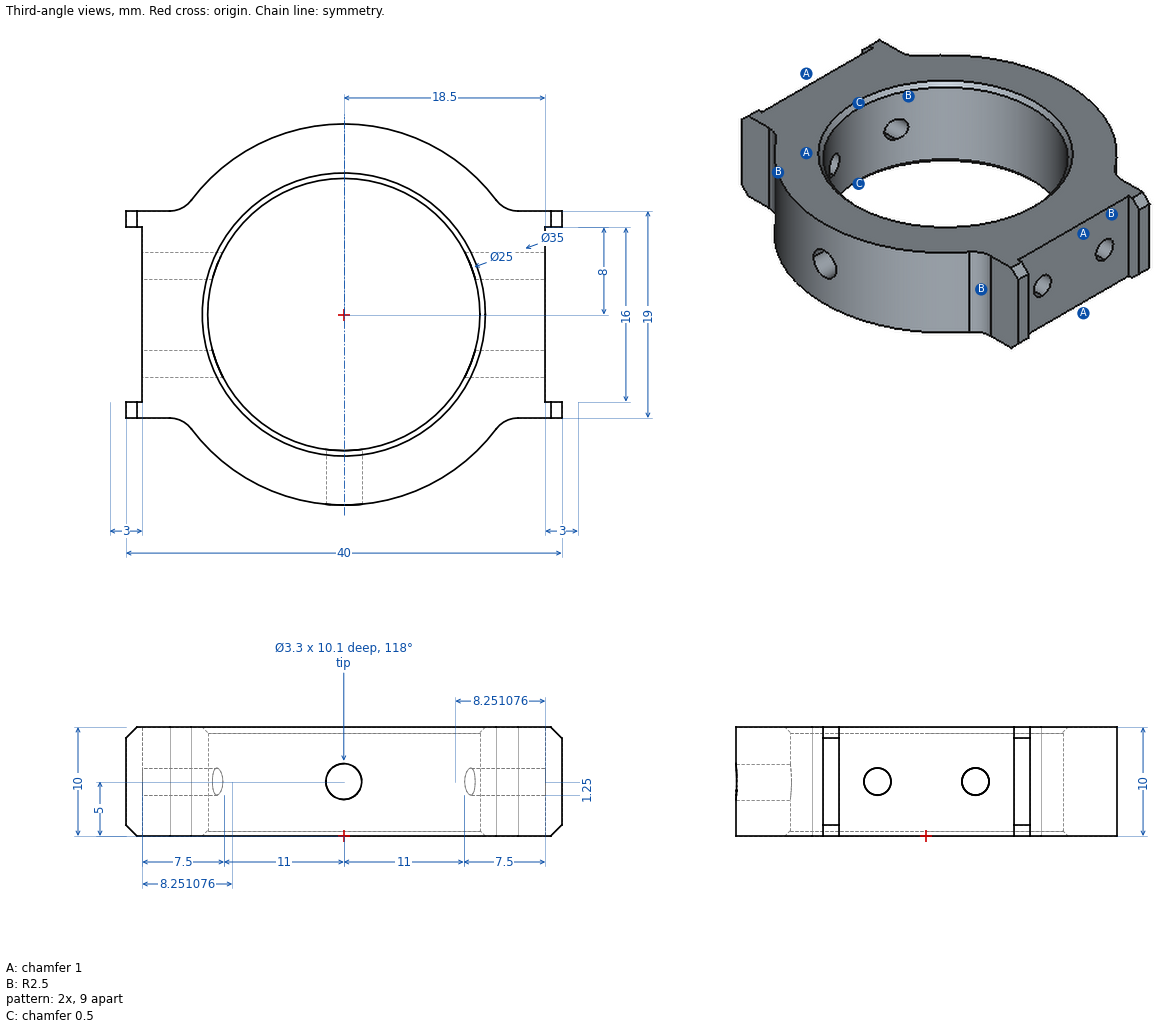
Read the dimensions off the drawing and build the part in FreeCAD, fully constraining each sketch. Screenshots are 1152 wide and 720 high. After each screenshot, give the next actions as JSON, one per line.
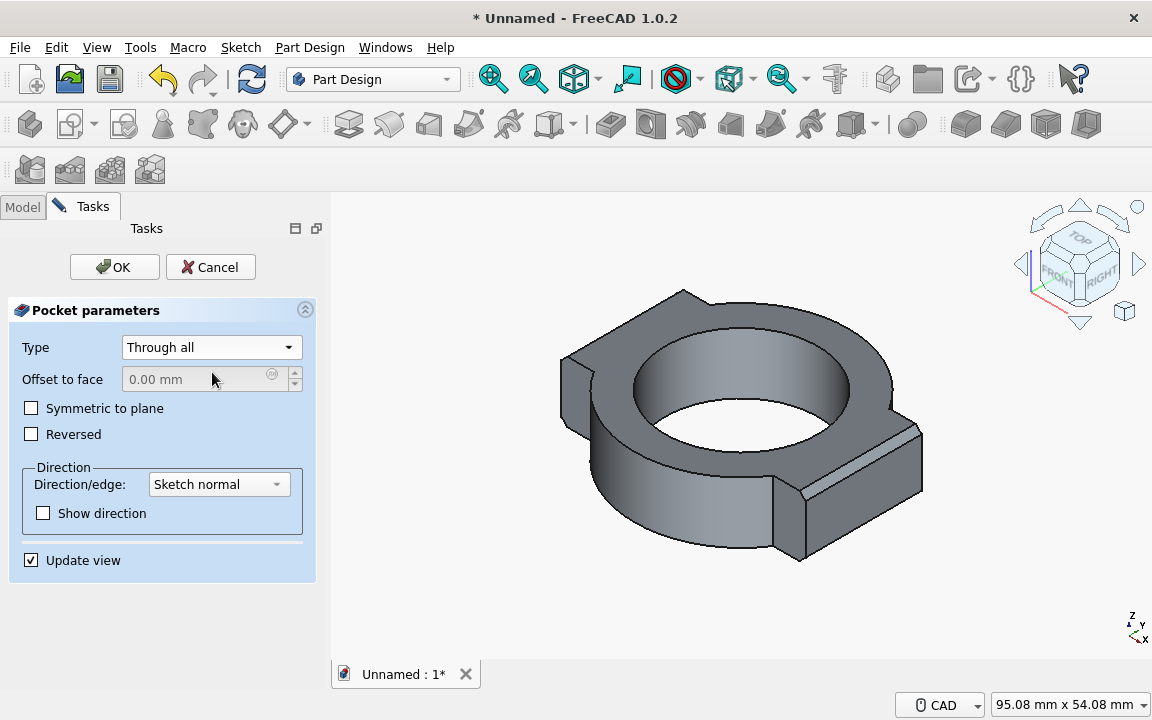
{"action": "left_click", "coordinate": [115, 267]}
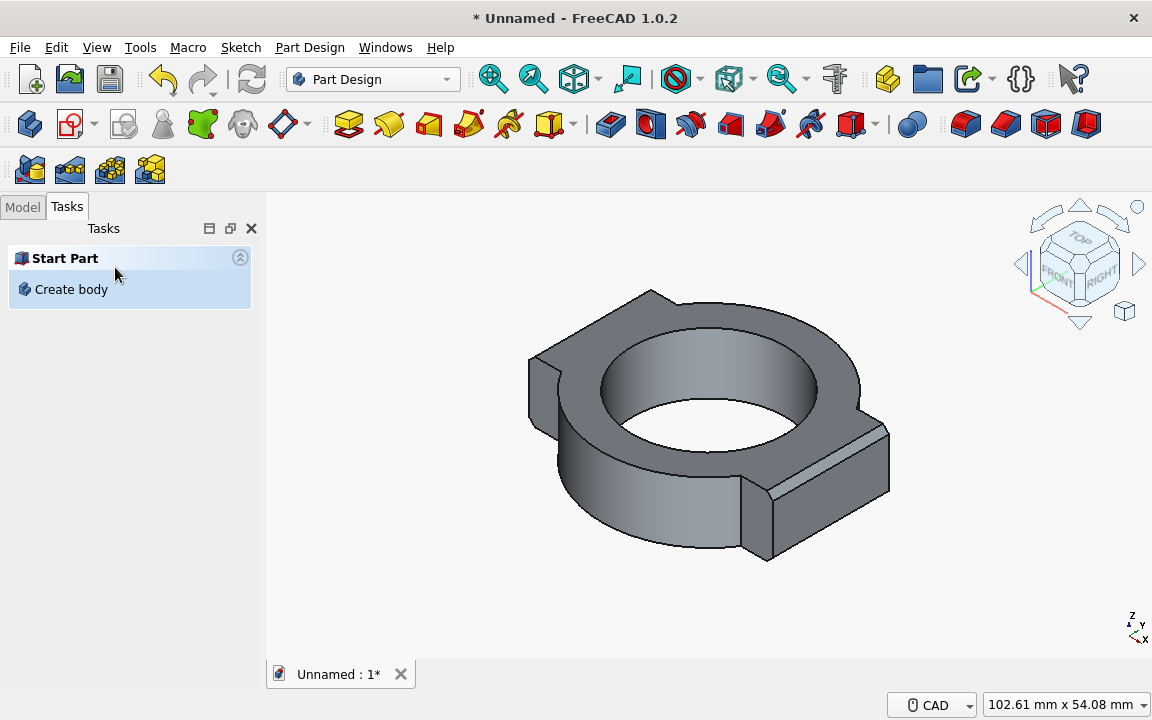
{"action": "left_click", "coordinate": [839, 429]}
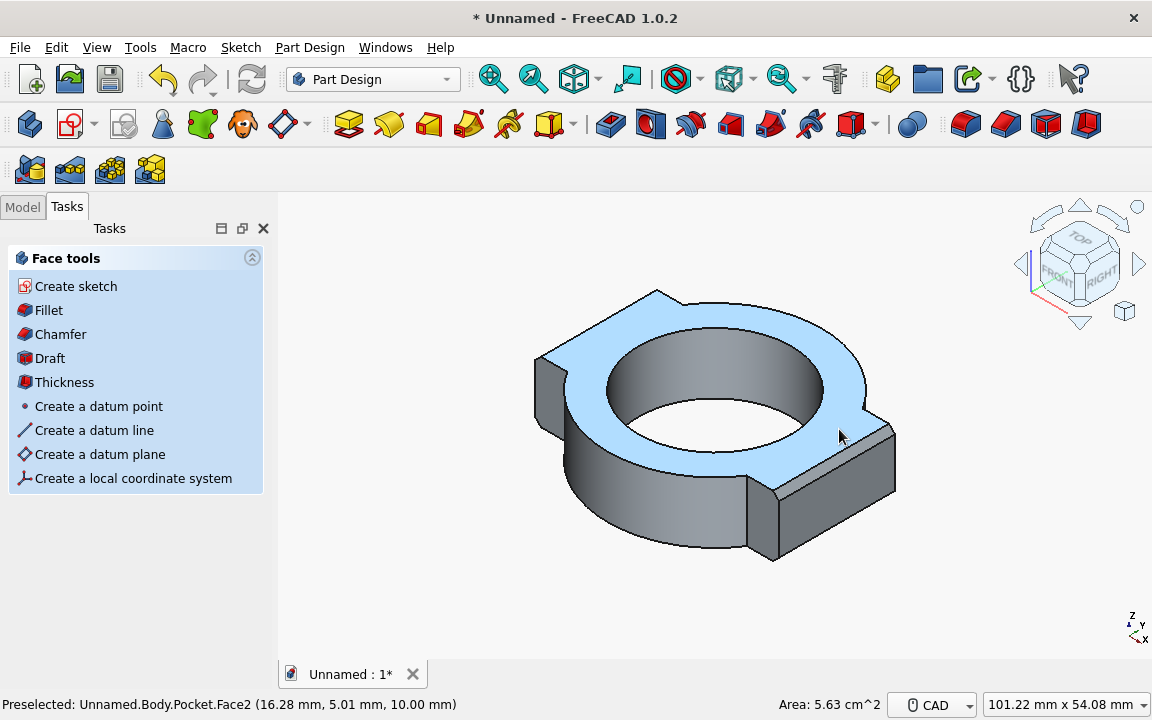
{"action": "left_click", "coordinate": [70, 124]}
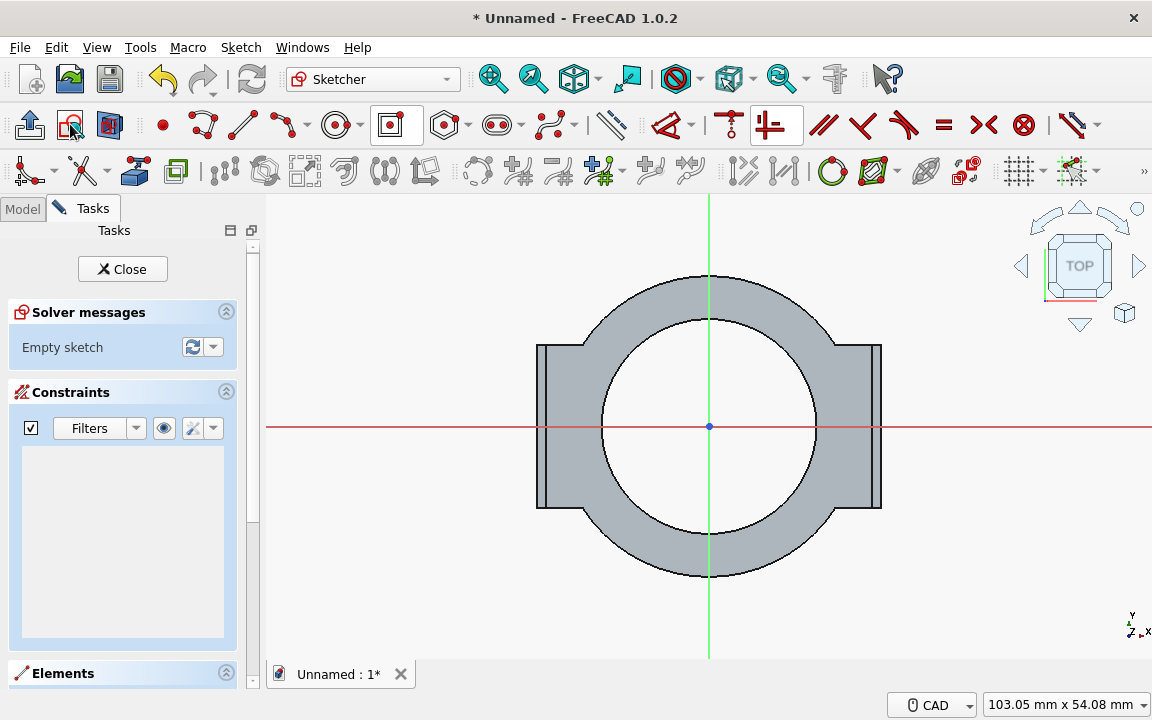
{"action": "left_click", "coordinate": [418, 126]}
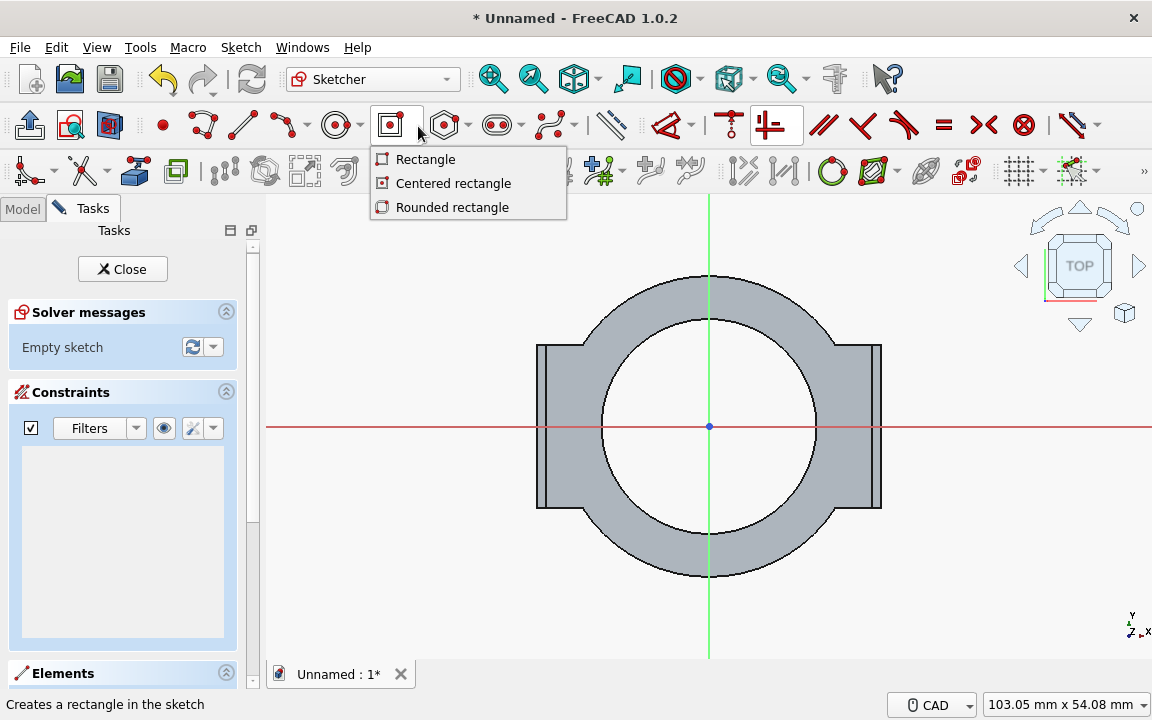
{"action": "left_click", "coordinate": [468, 159]}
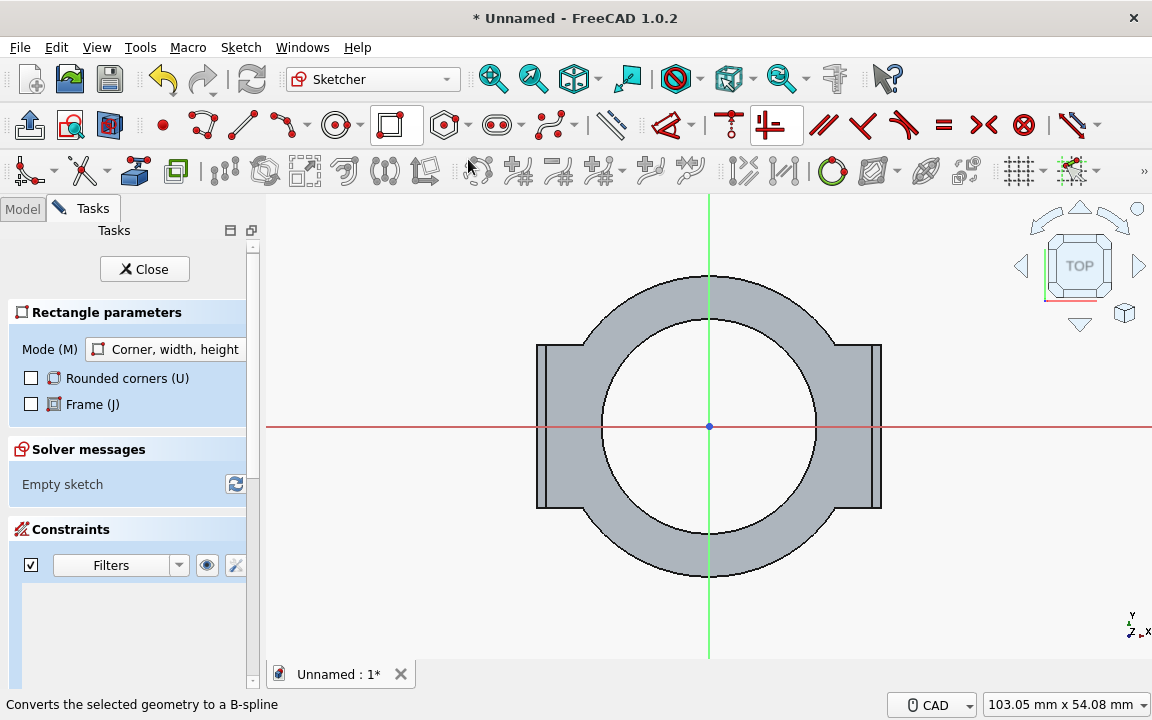
{"action": "left_click", "coordinate": [868, 358]}
{"action": "mouse_move", "coordinate": [894, 495]}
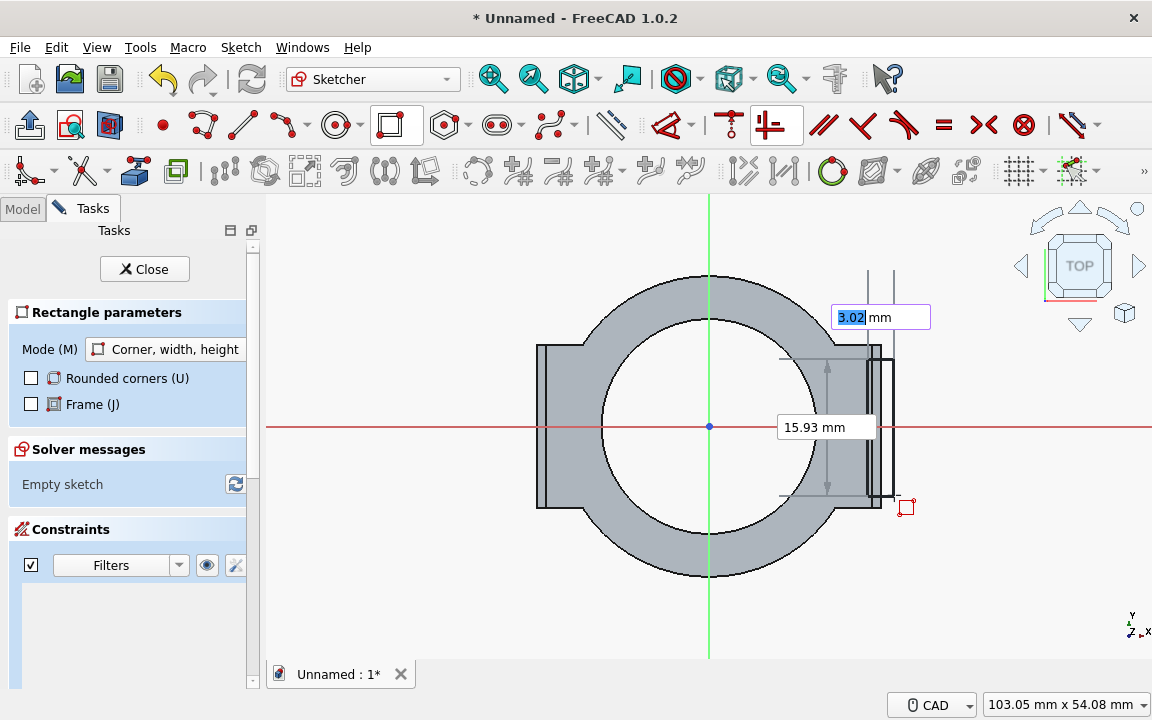
{"action": "type", "text": "3"}
{"action": "key", "text": "Tab"}
{"action": "type", "text": "16"}
{"action": "key", "text": "Return"}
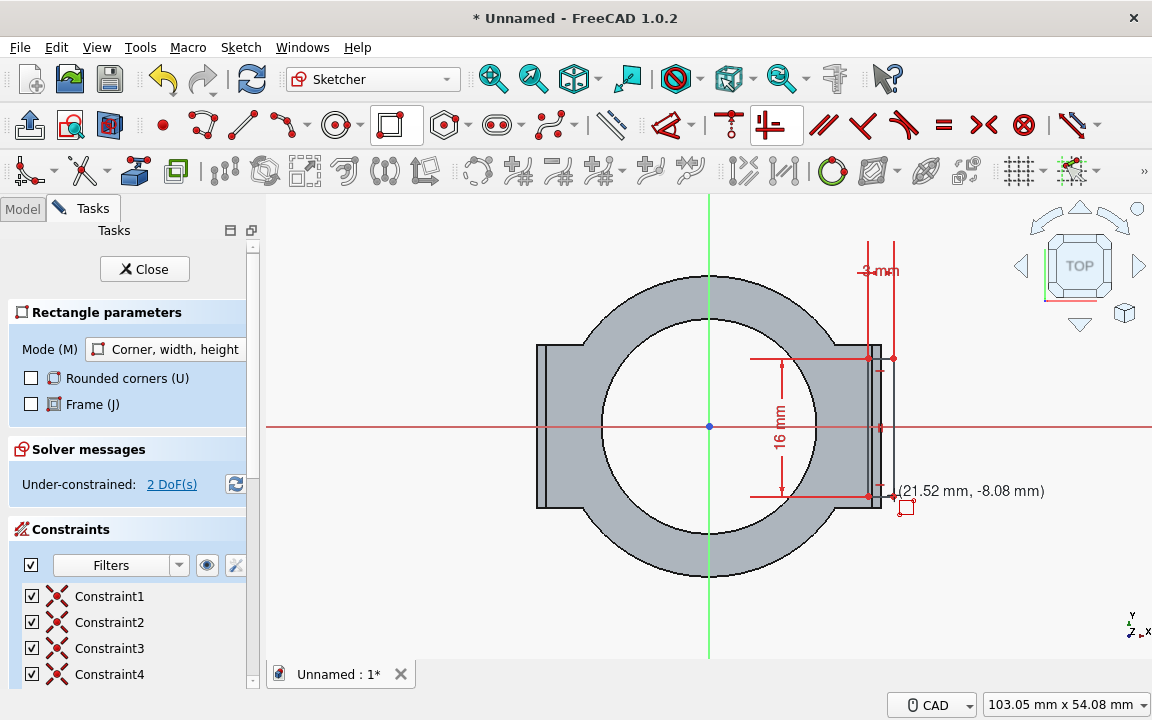
{"action": "left_click", "coordinate": [524, 358]}
{"action": "mouse_move", "coordinate": [550, 495]}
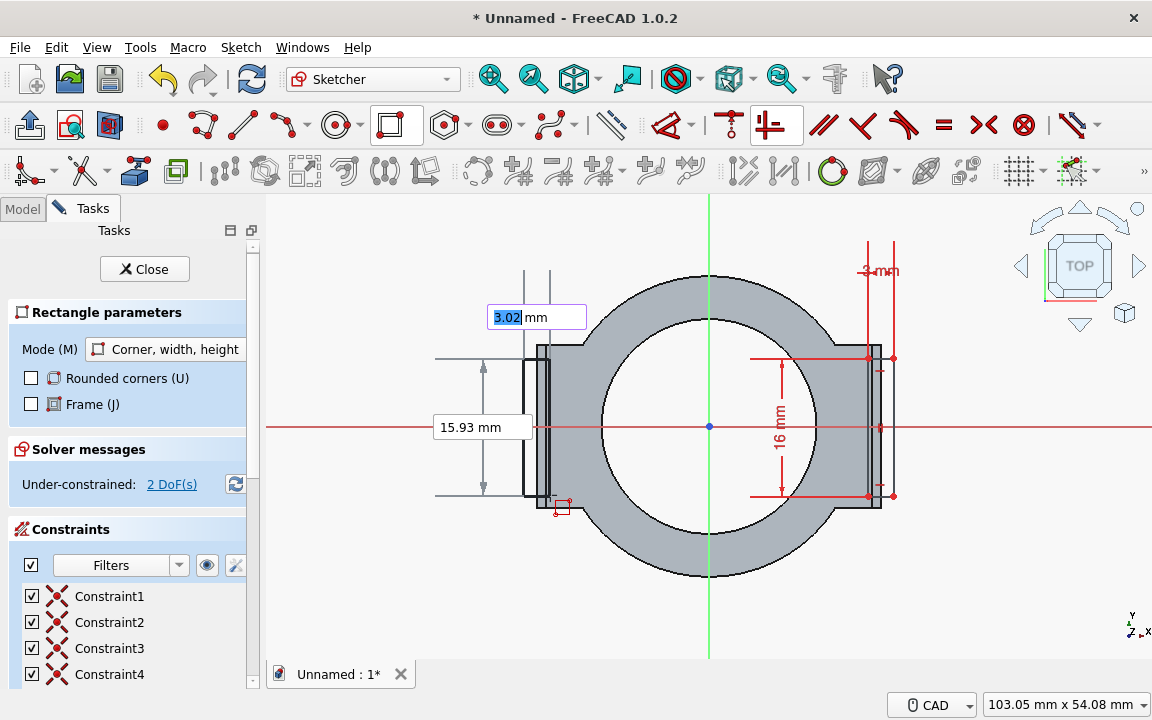
{"action": "type", "text": "3"}
{"action": "key", "text": "Tab"}
{"action": "type", "text": "16"}
{"action": "key", "text": "Return"}
{"action": "key", "text": "Escape"}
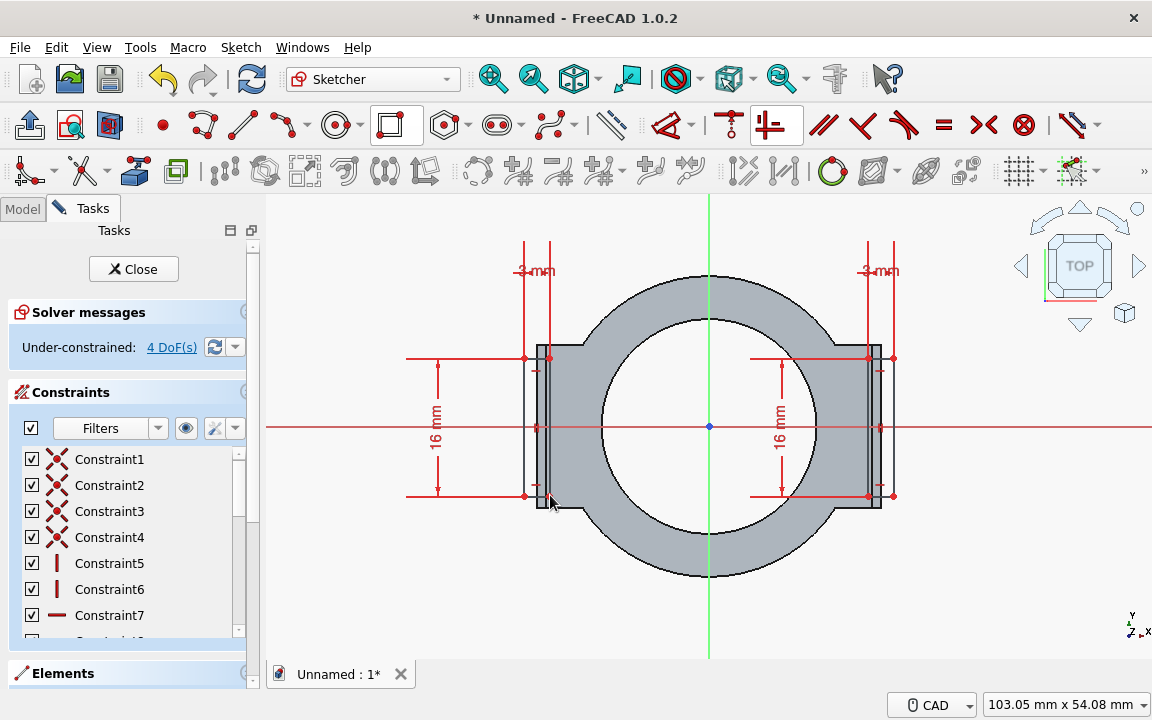
{"action": "left_click", "coordinate": [894, 359]}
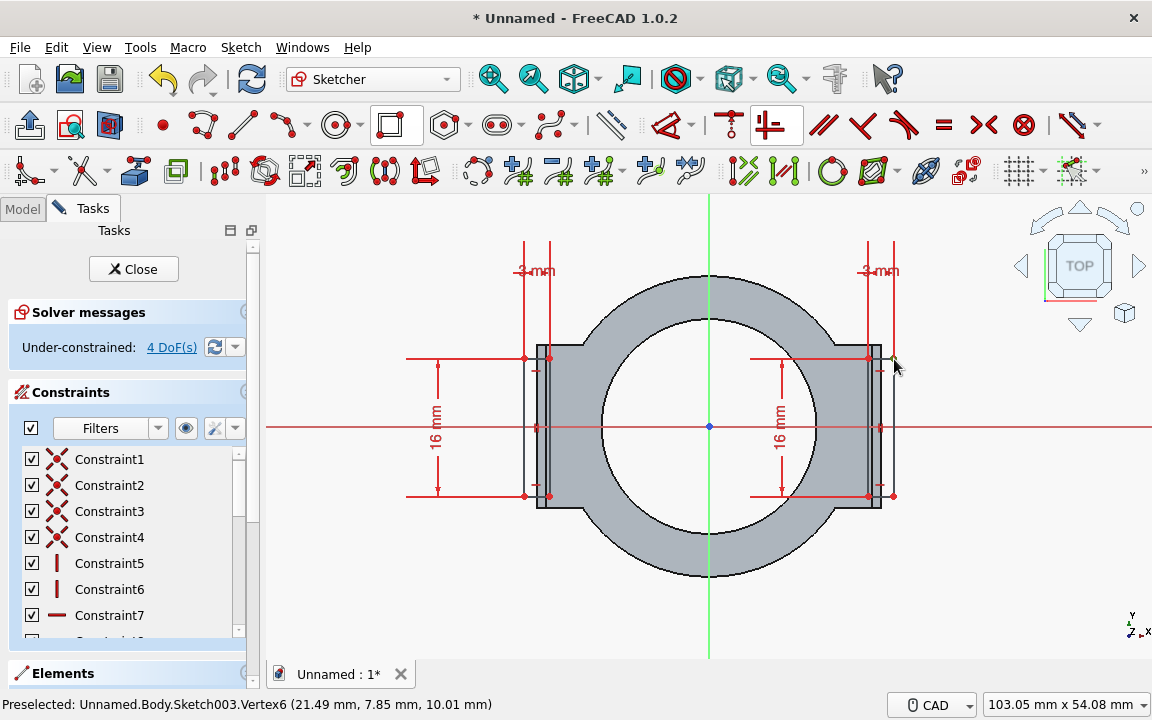
{"action": "left_click", "coordinate": [524, 359]}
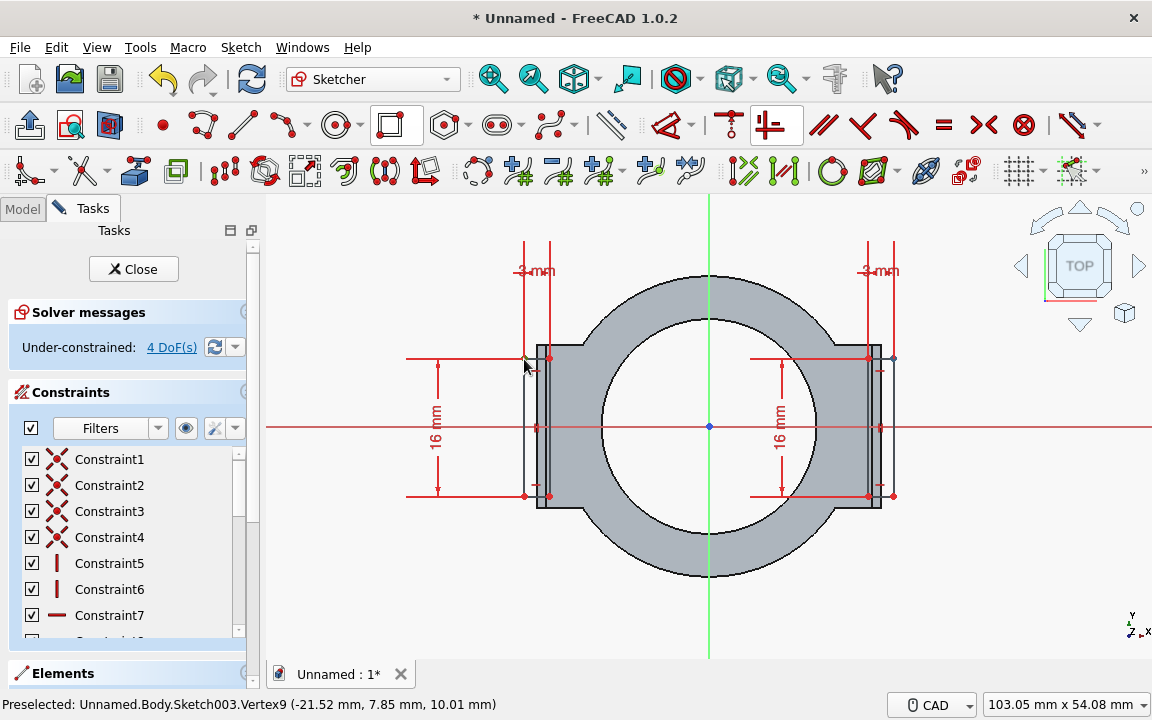
{"action": "left_click", "coordinate": [709, 602]}